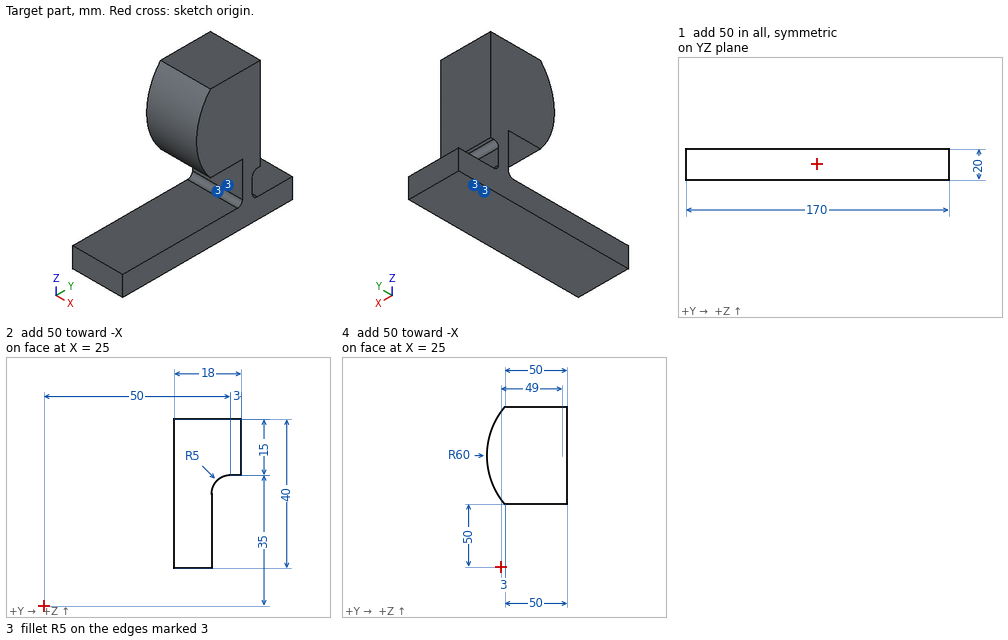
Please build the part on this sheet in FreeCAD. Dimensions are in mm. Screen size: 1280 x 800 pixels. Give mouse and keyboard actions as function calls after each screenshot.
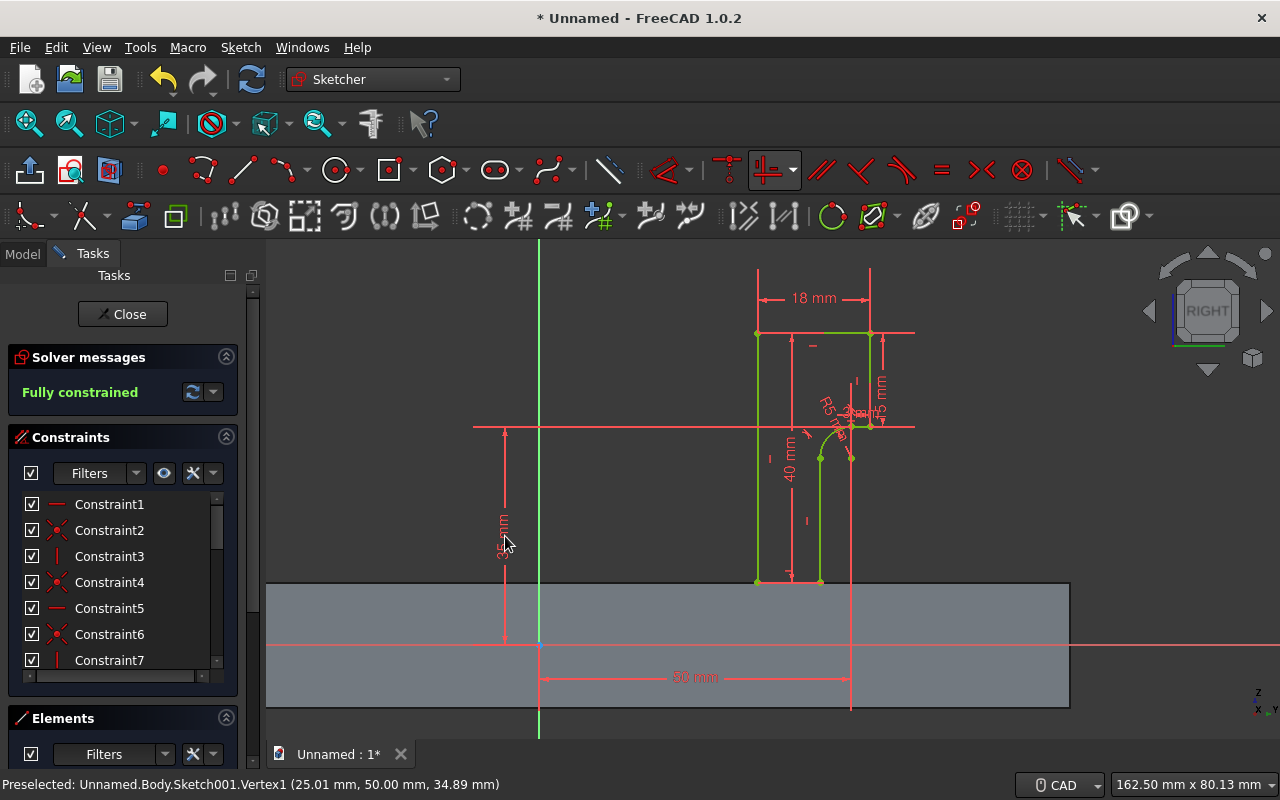
click(123, 314)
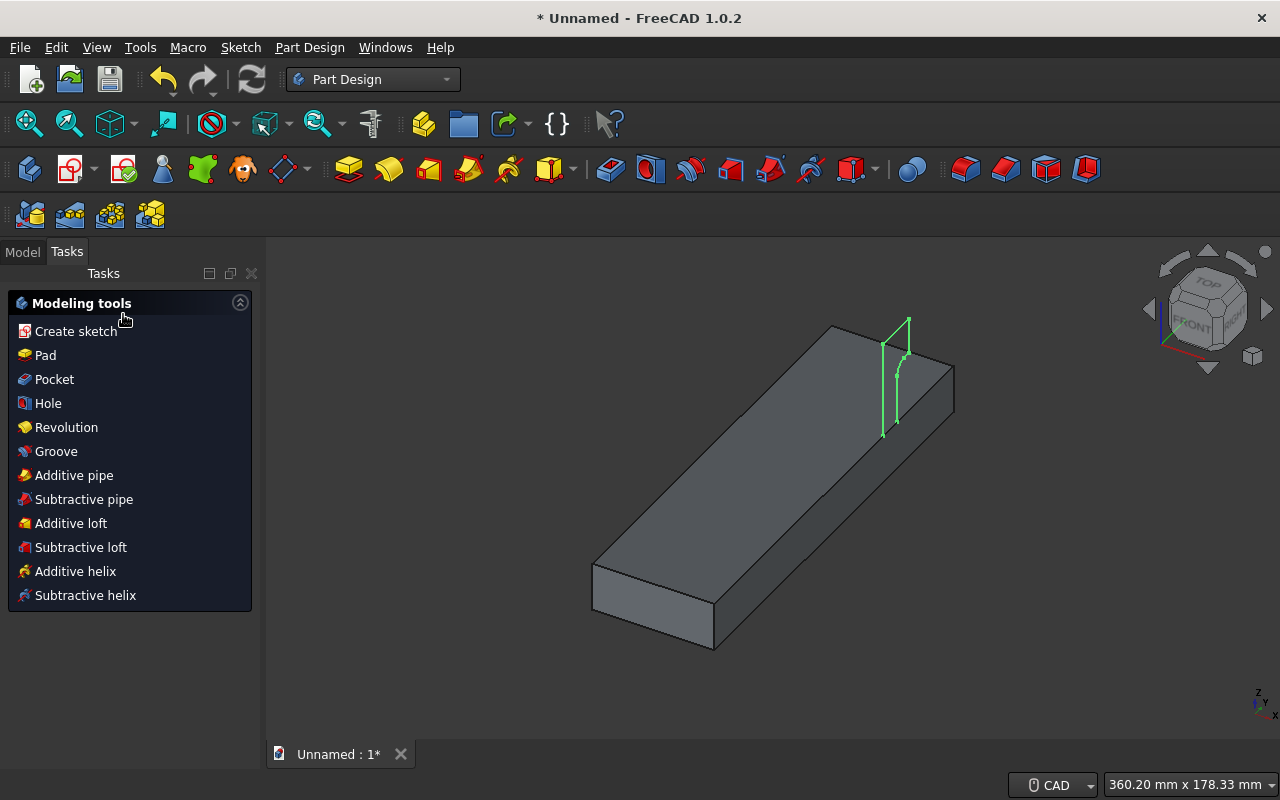
click(350, 170)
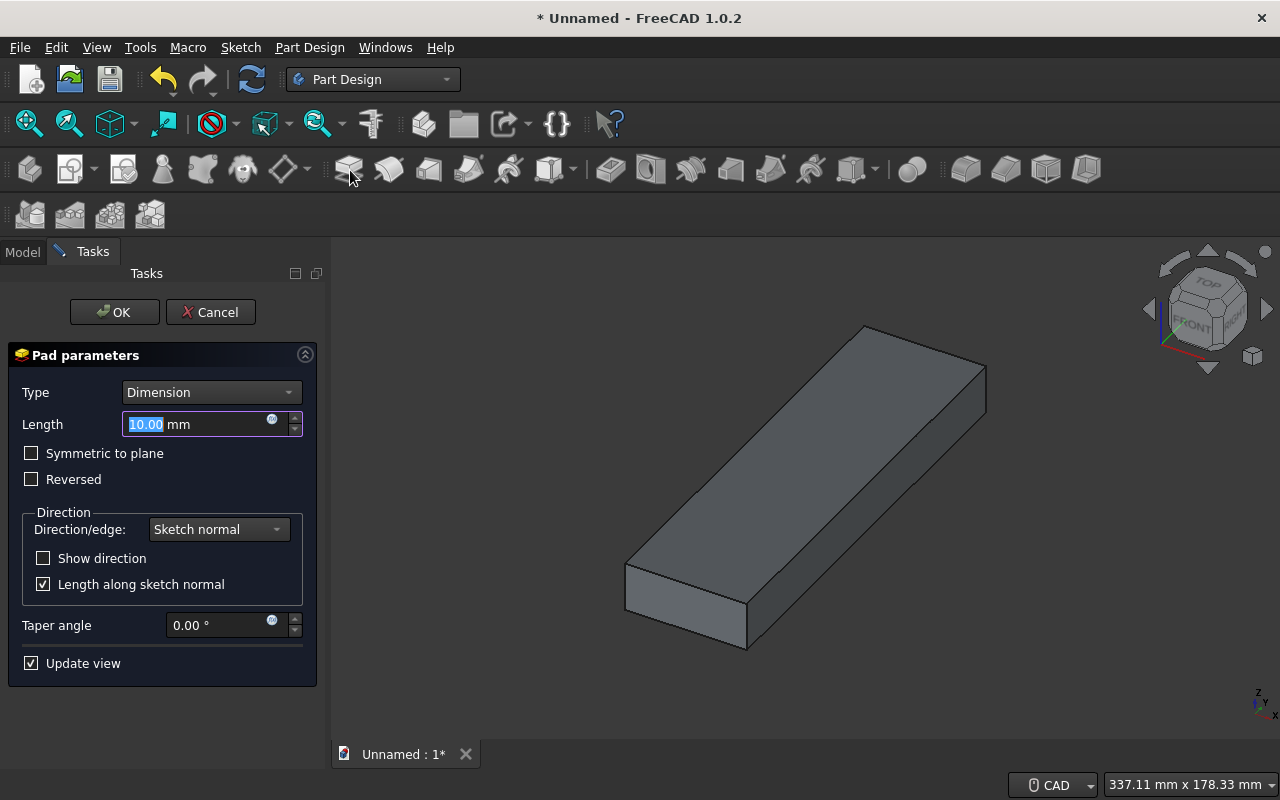
text(50)
key(Tab)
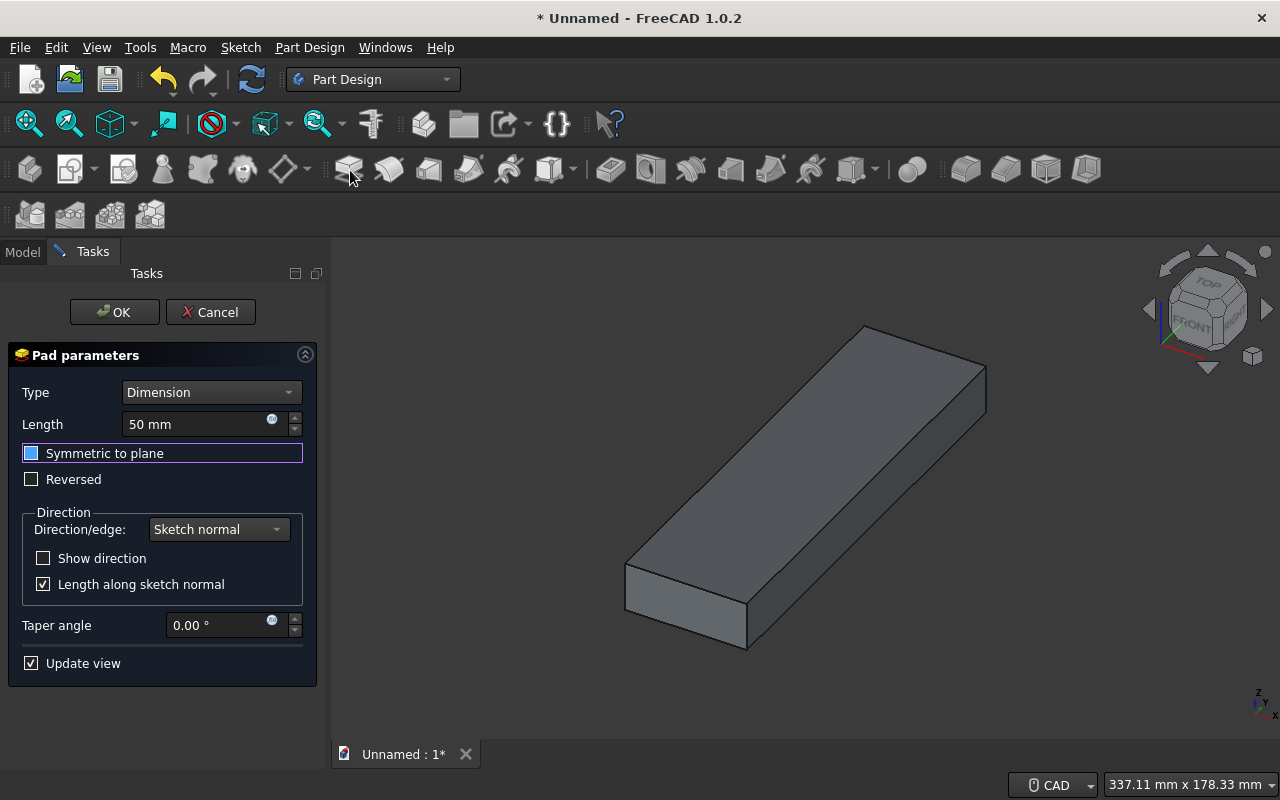
click(30, 479)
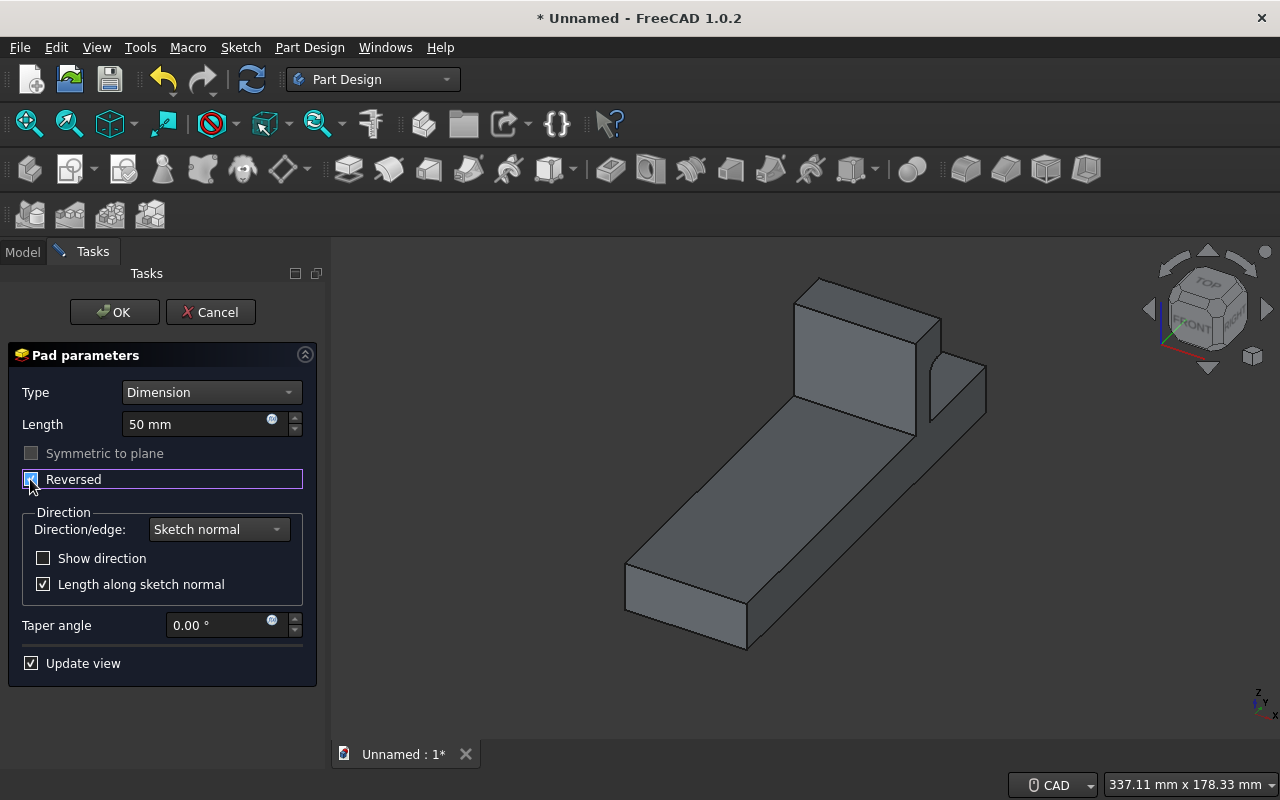
click(115, 312)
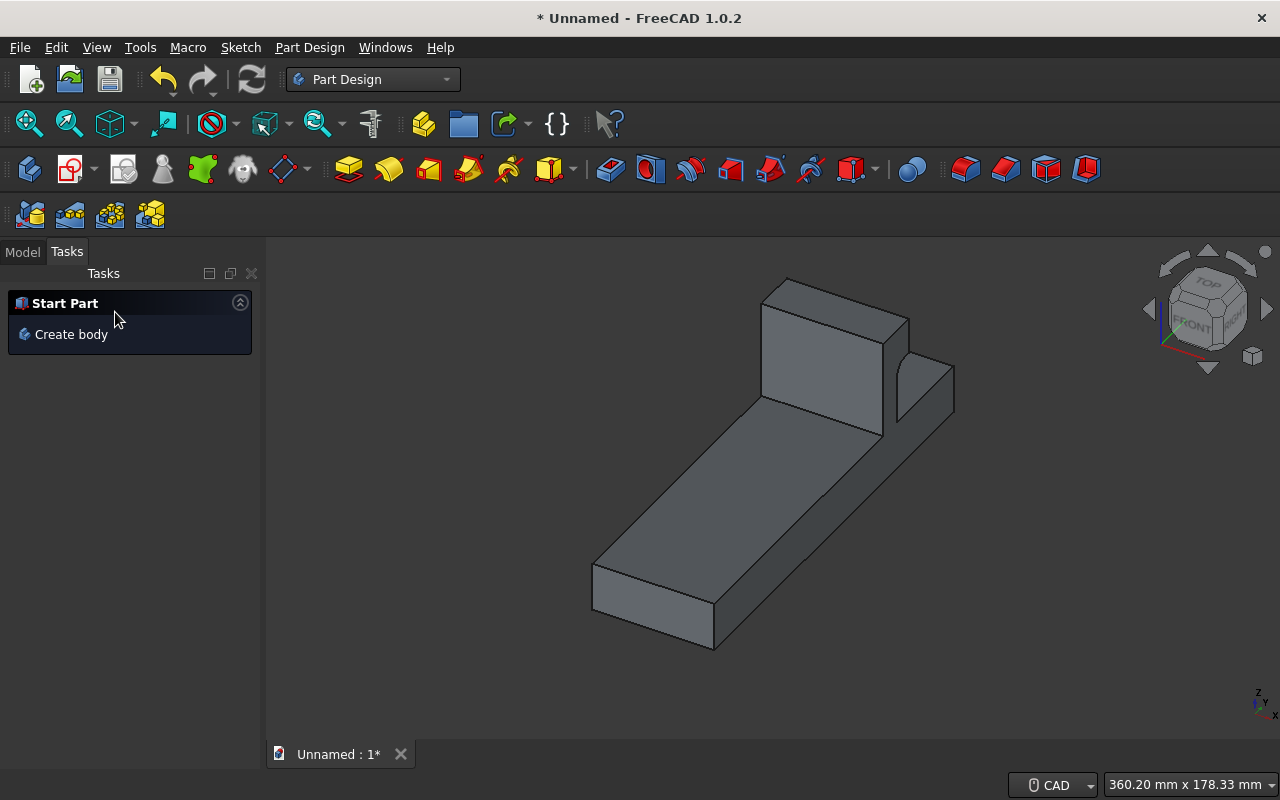
key(v)
key(f)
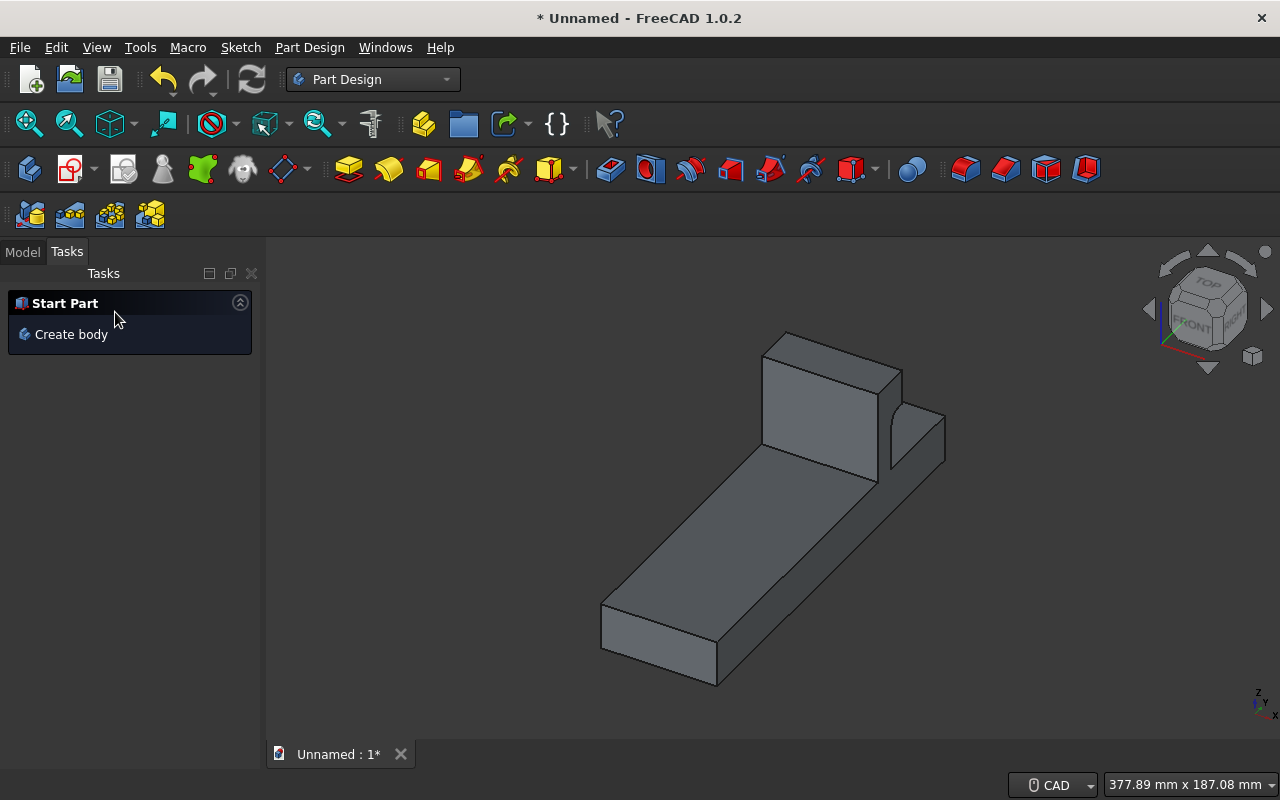
key(0)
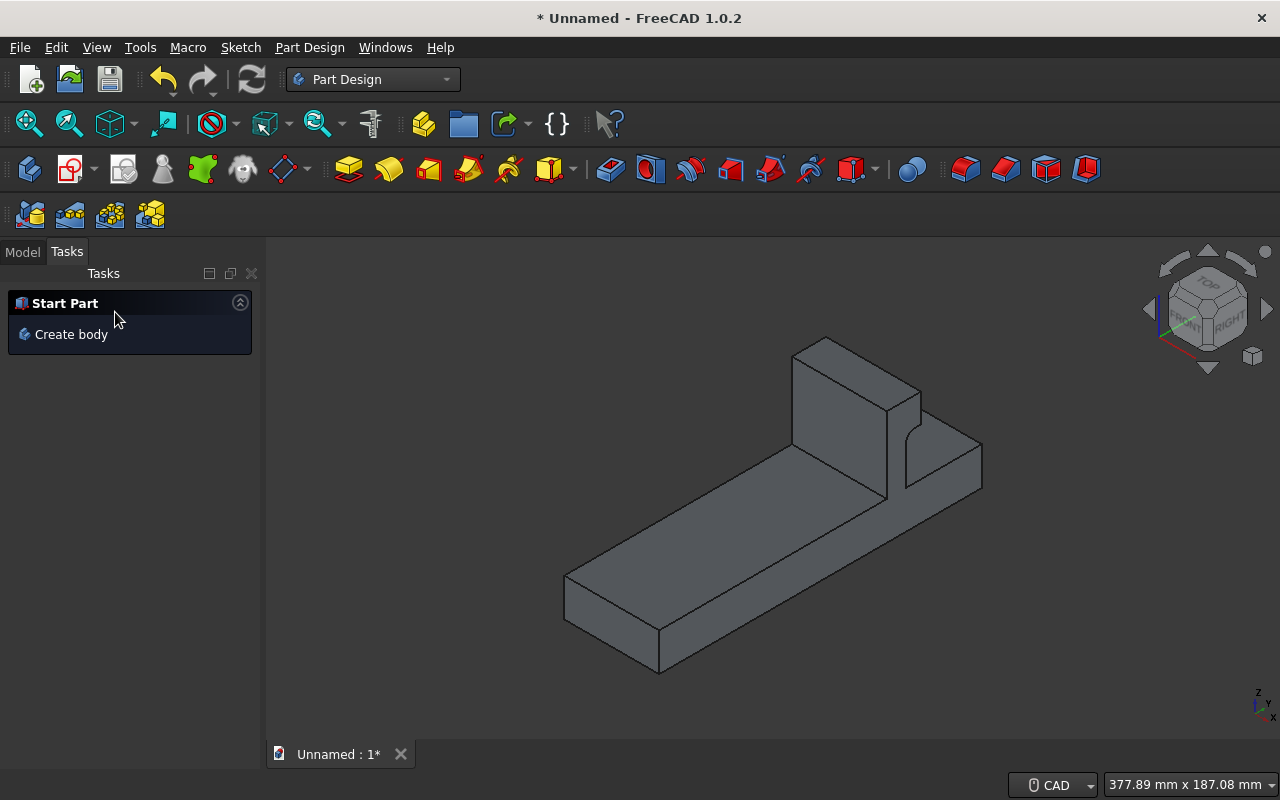
key(2)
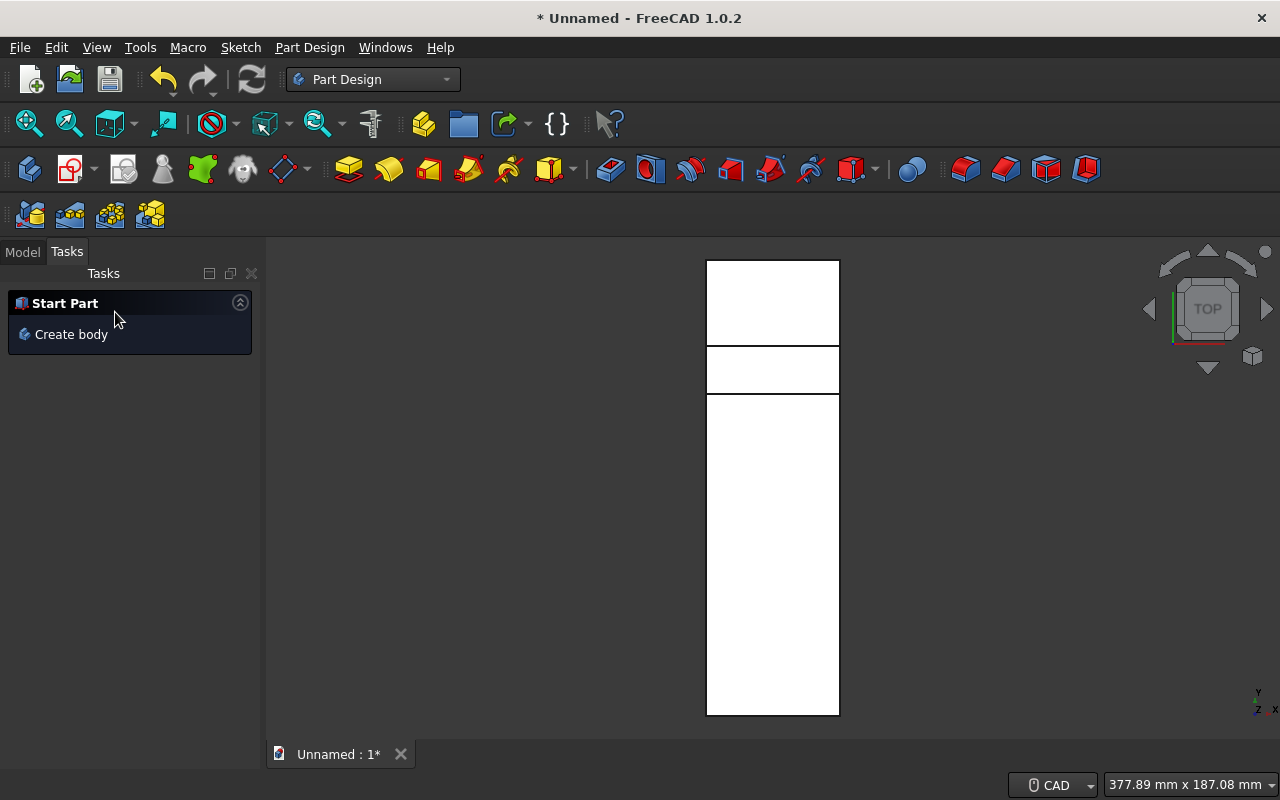
key(1)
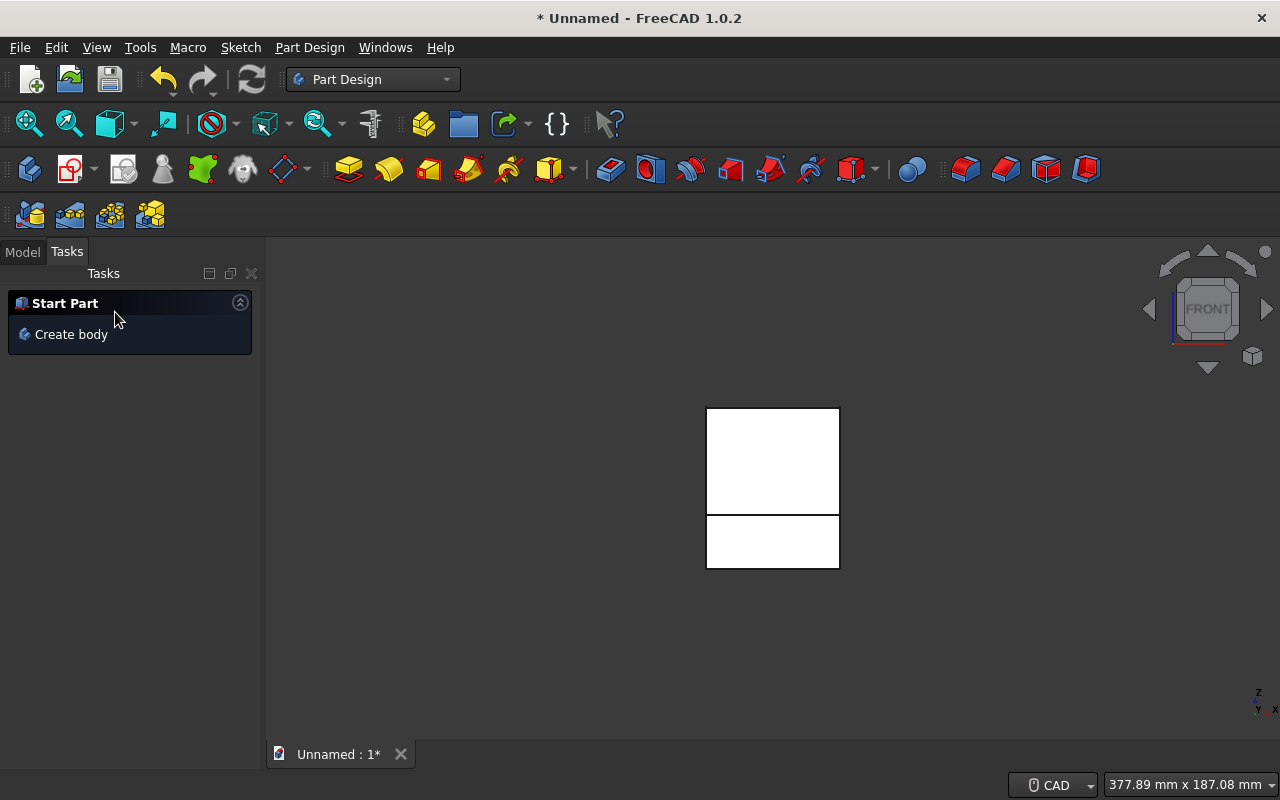
key(v)
key(f)